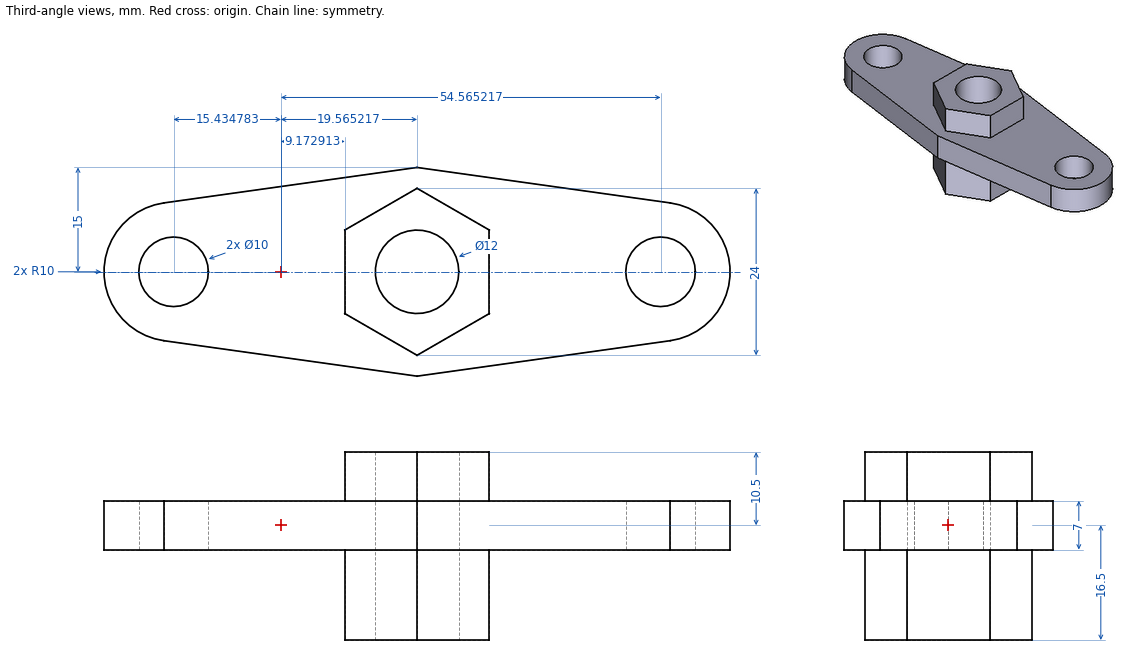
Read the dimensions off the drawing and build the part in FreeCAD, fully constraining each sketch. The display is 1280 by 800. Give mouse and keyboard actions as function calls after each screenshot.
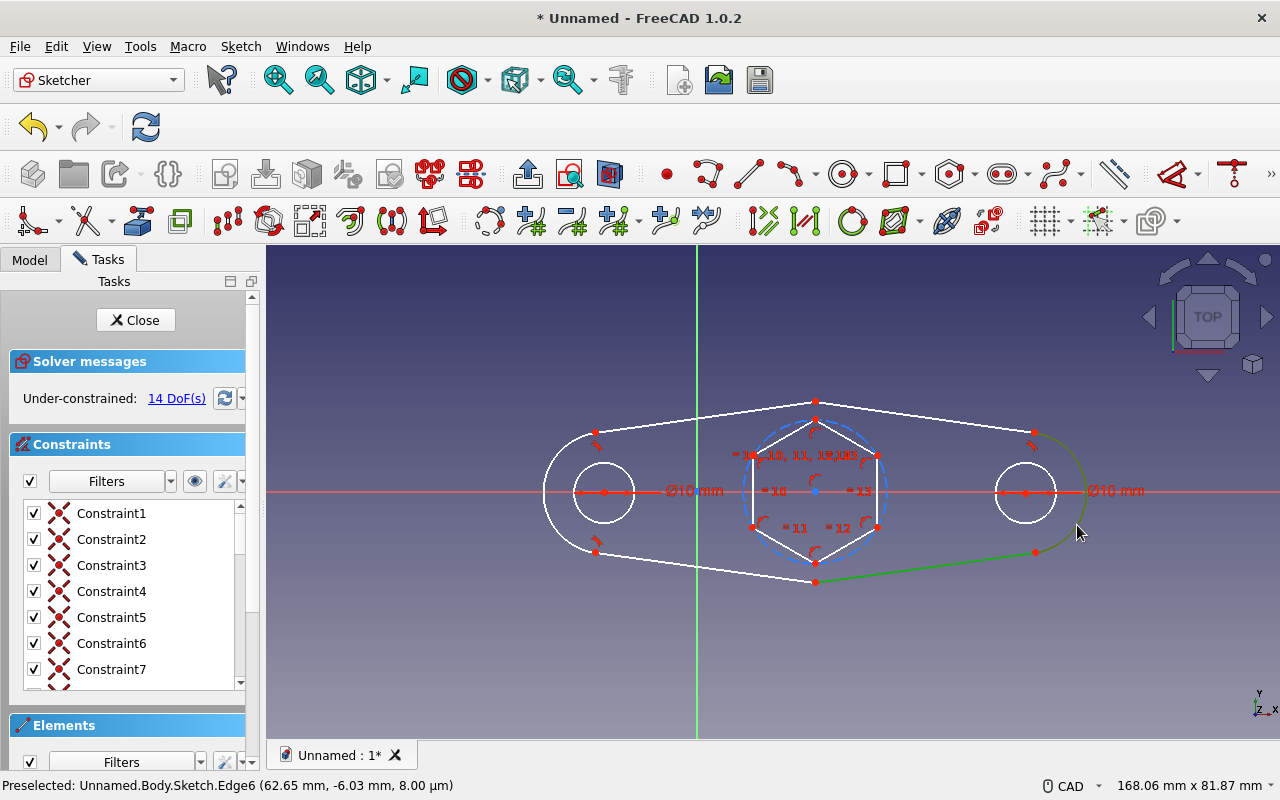
key(t)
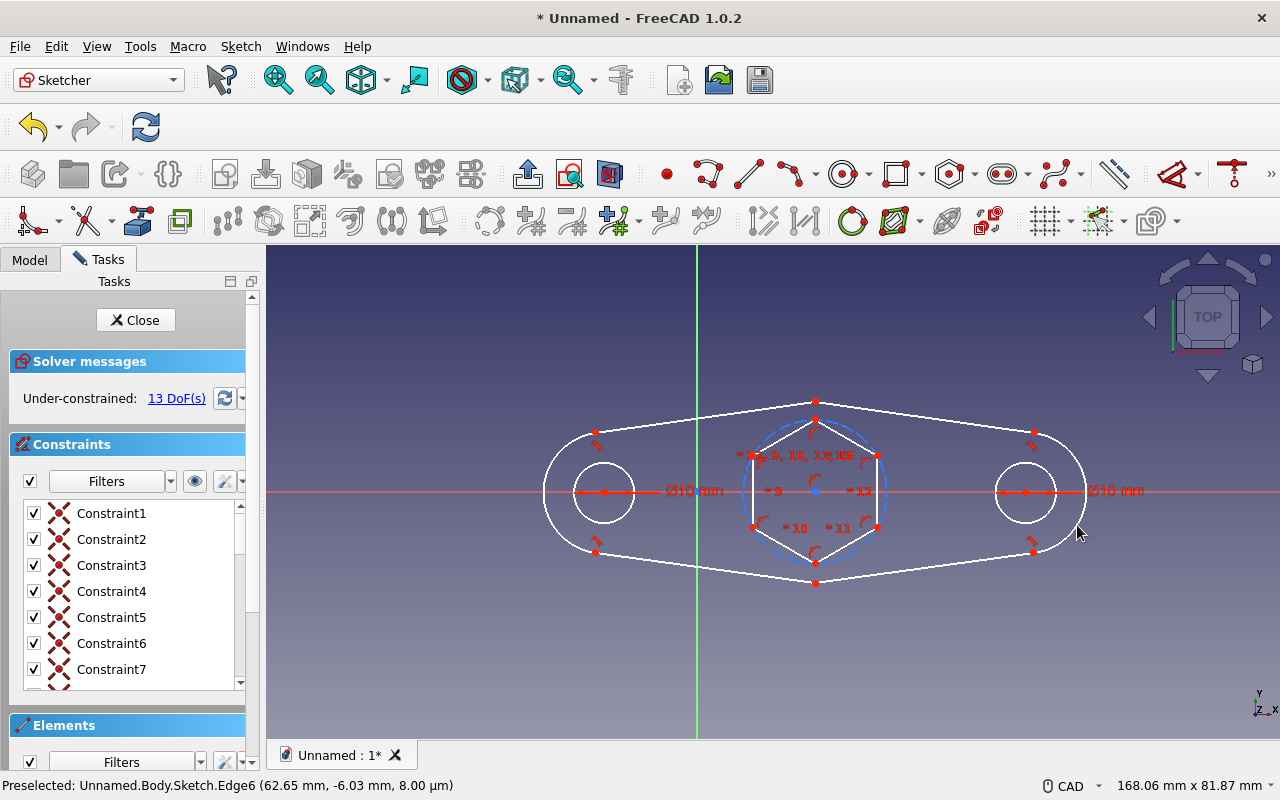
scroll(753, 492, up, 2)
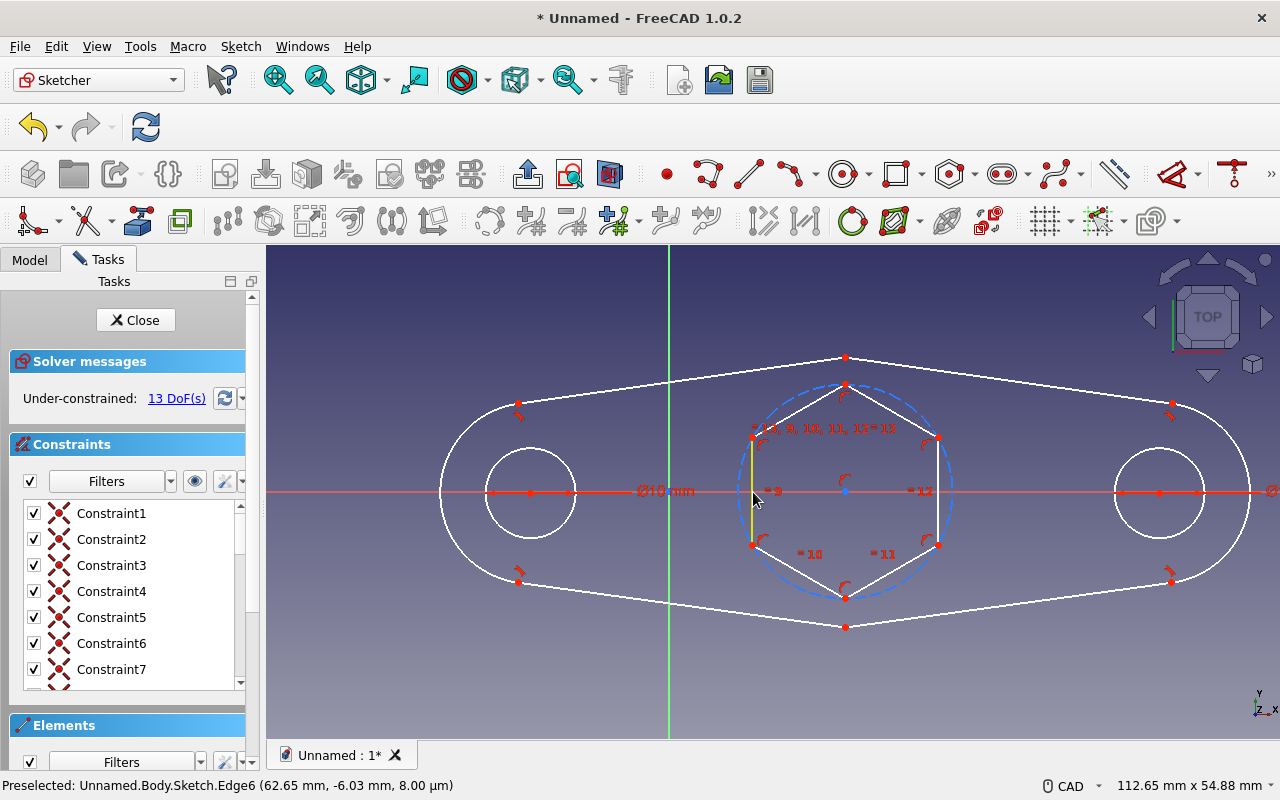
click(752, 492)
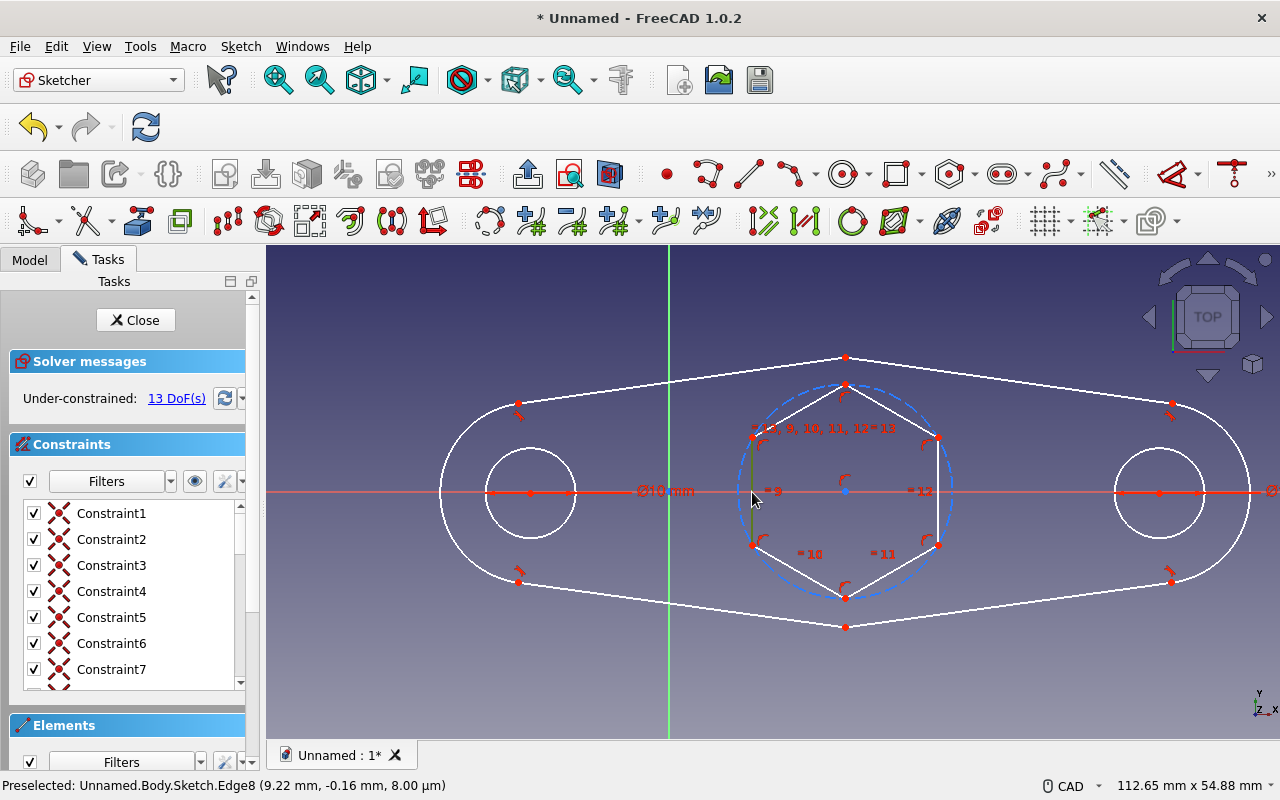
key(v)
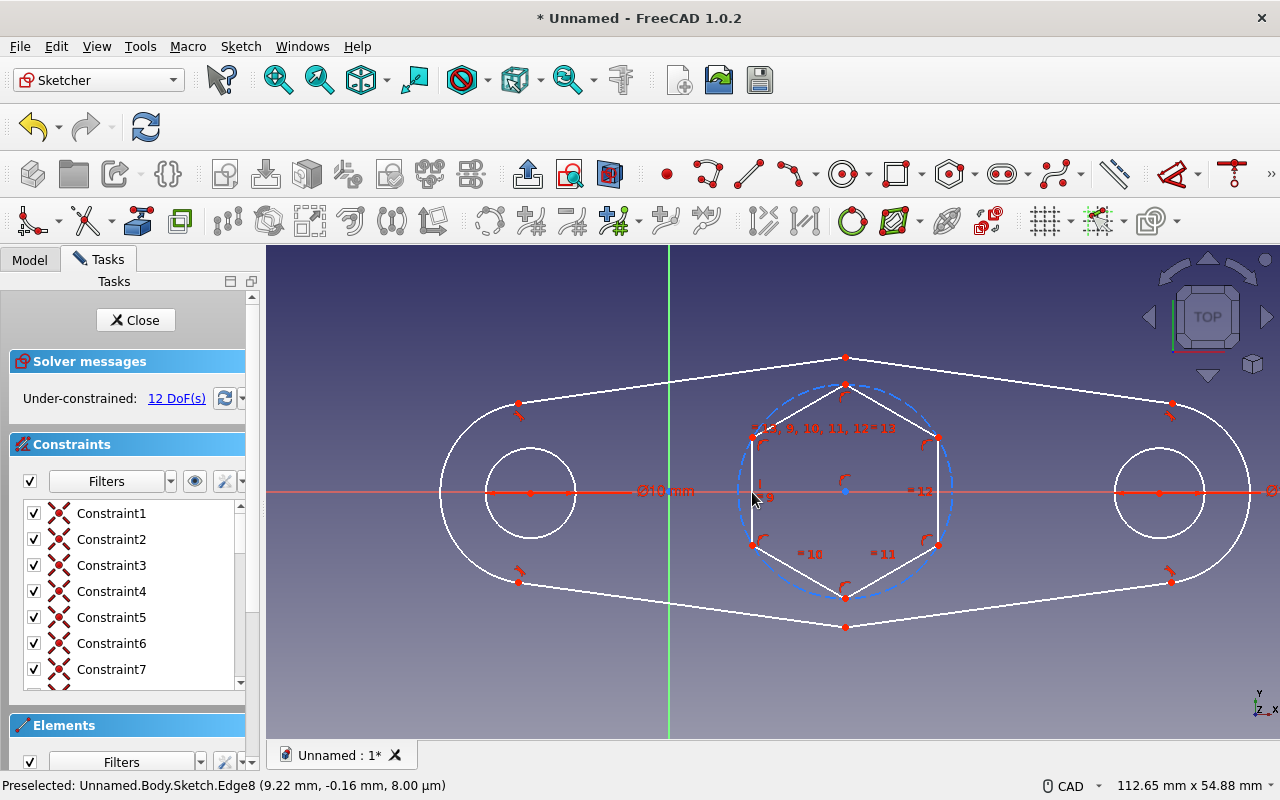
click(455, 444)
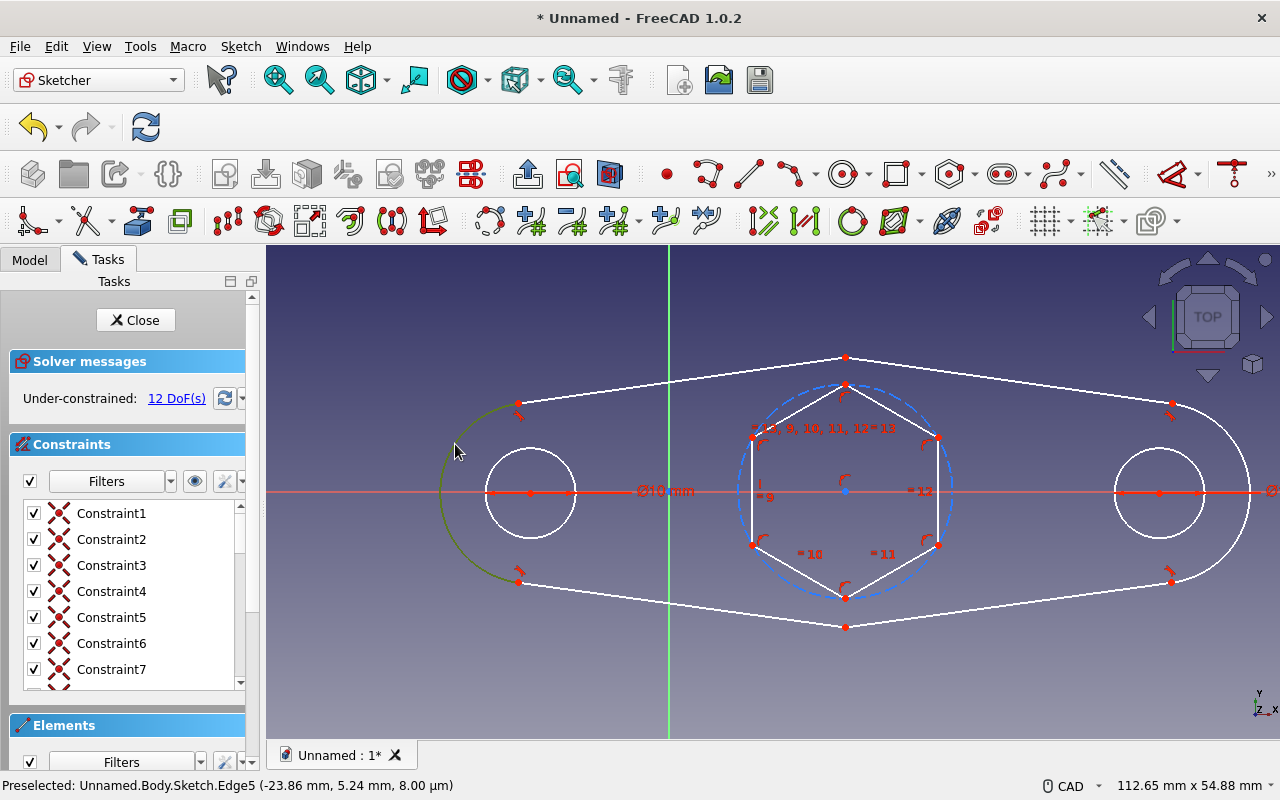
scroll(418, 493, down, 2)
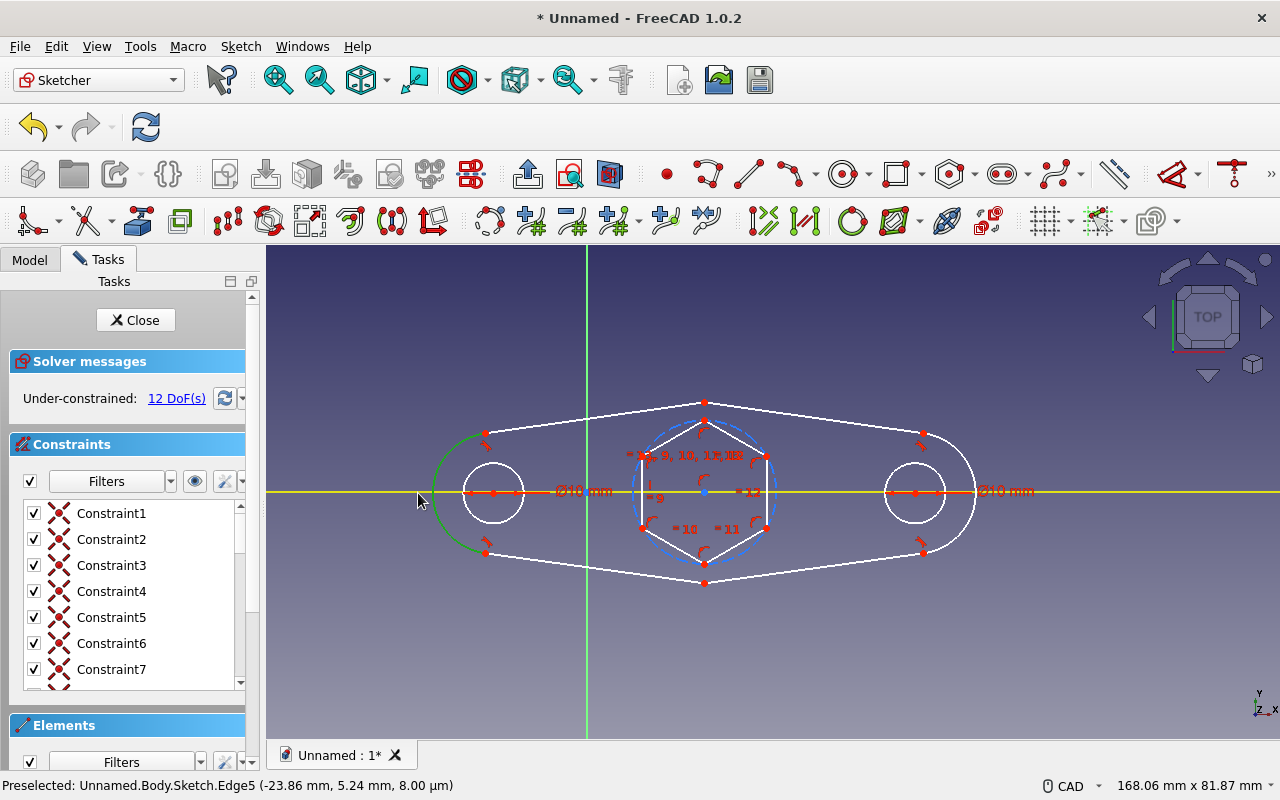
click(966, 526)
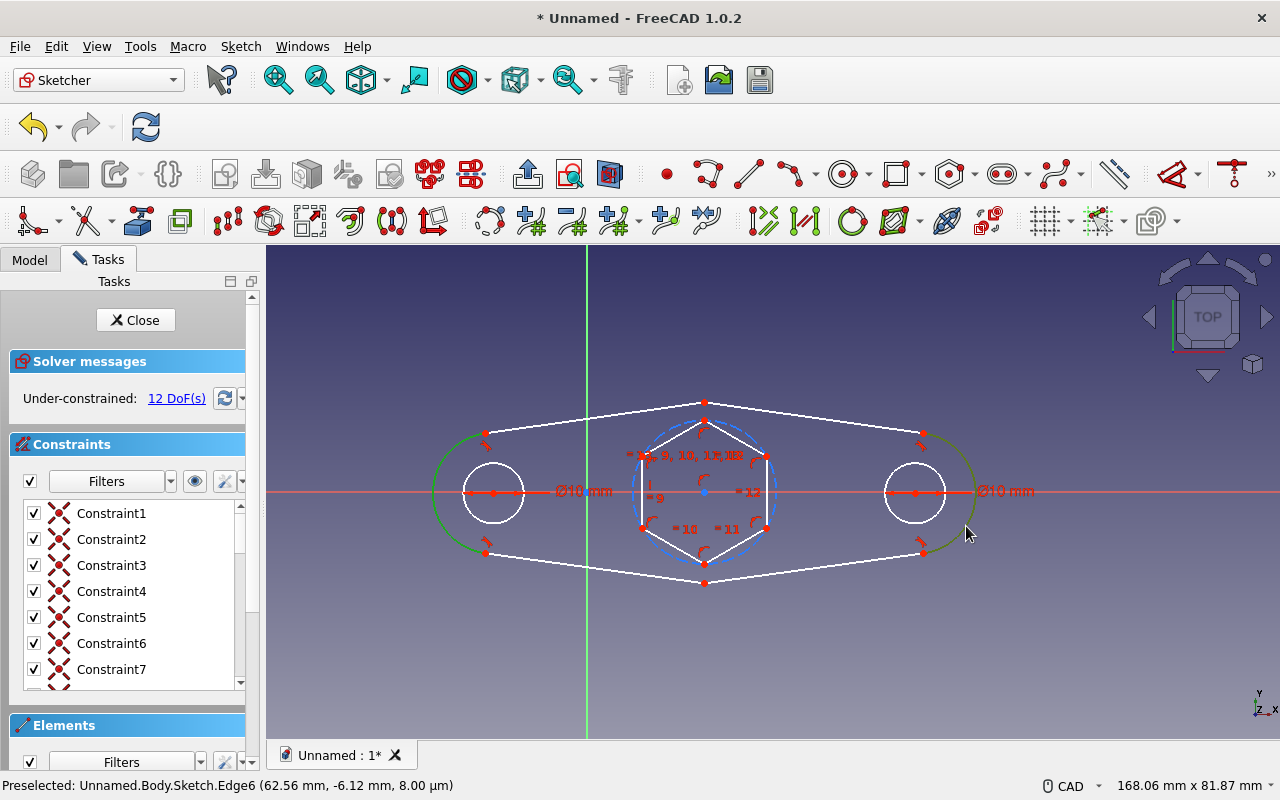
key(e)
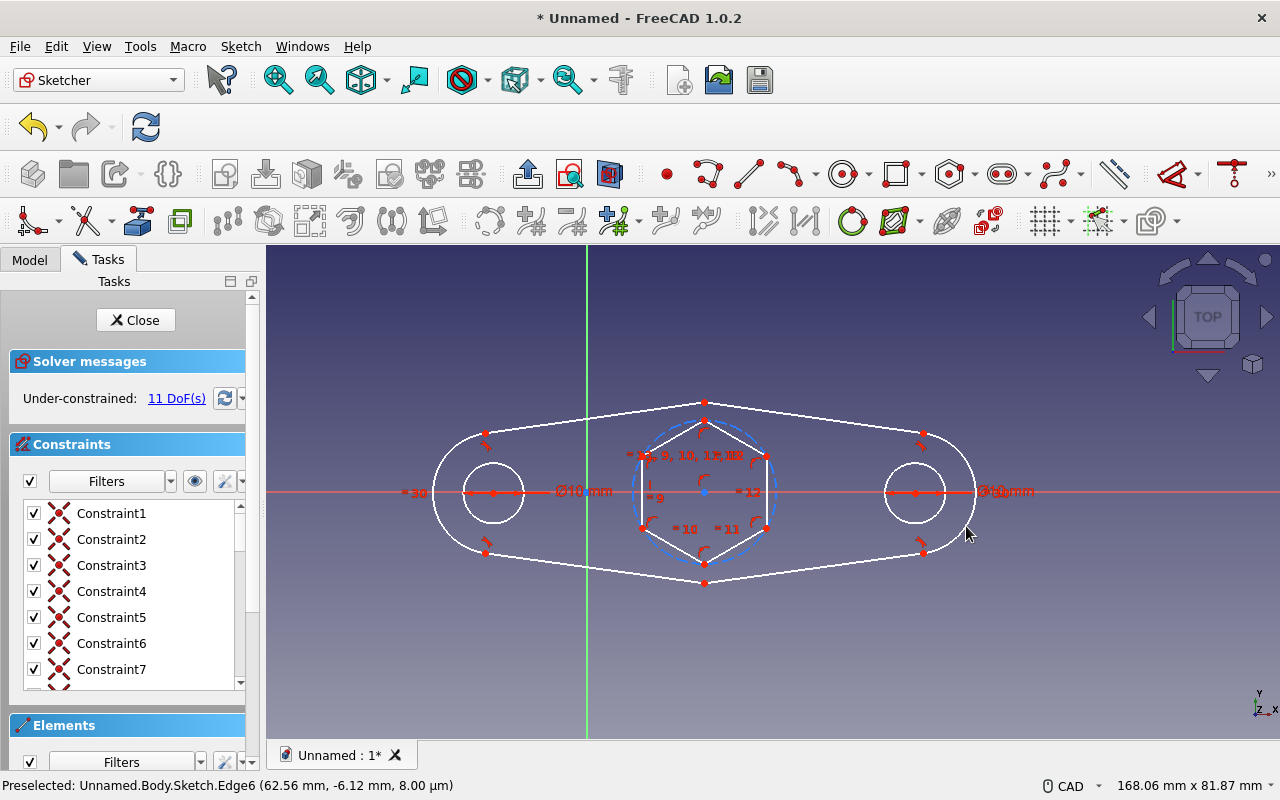
click(494, 493)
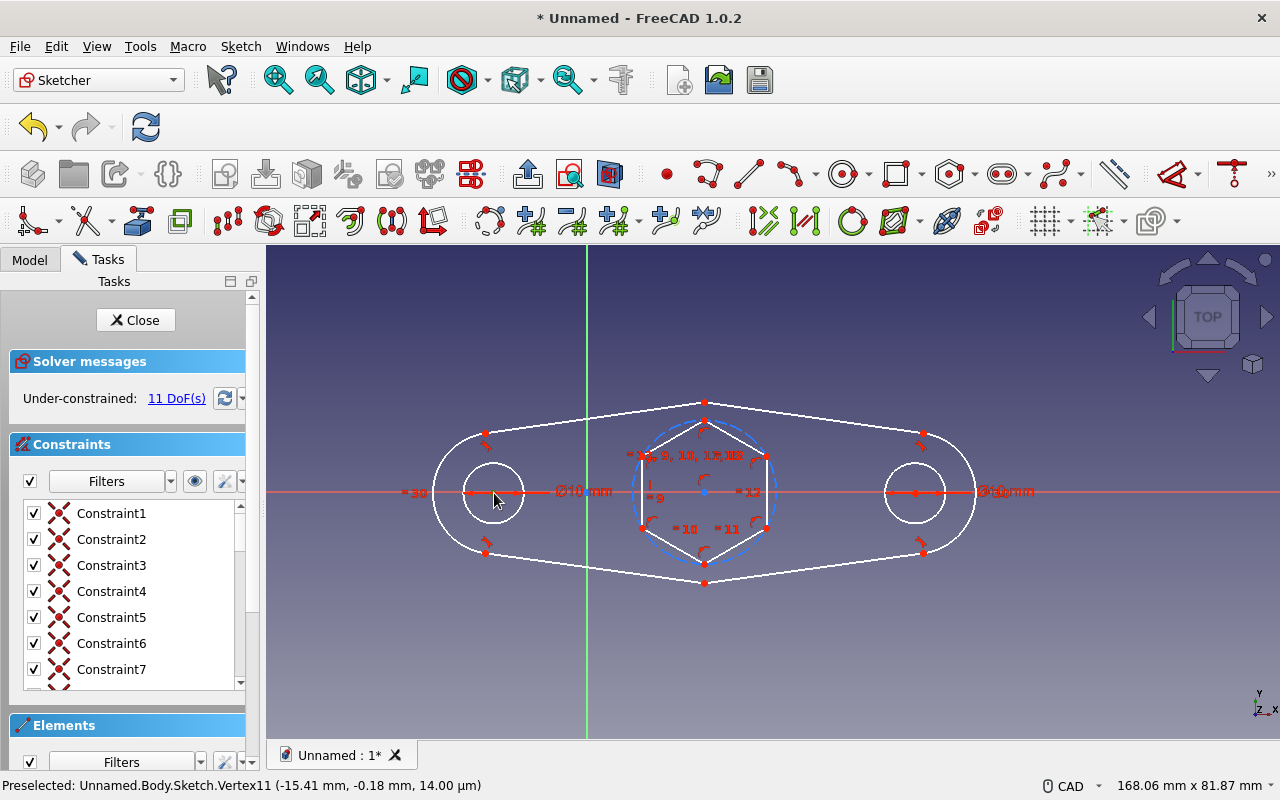
click(353, 492)